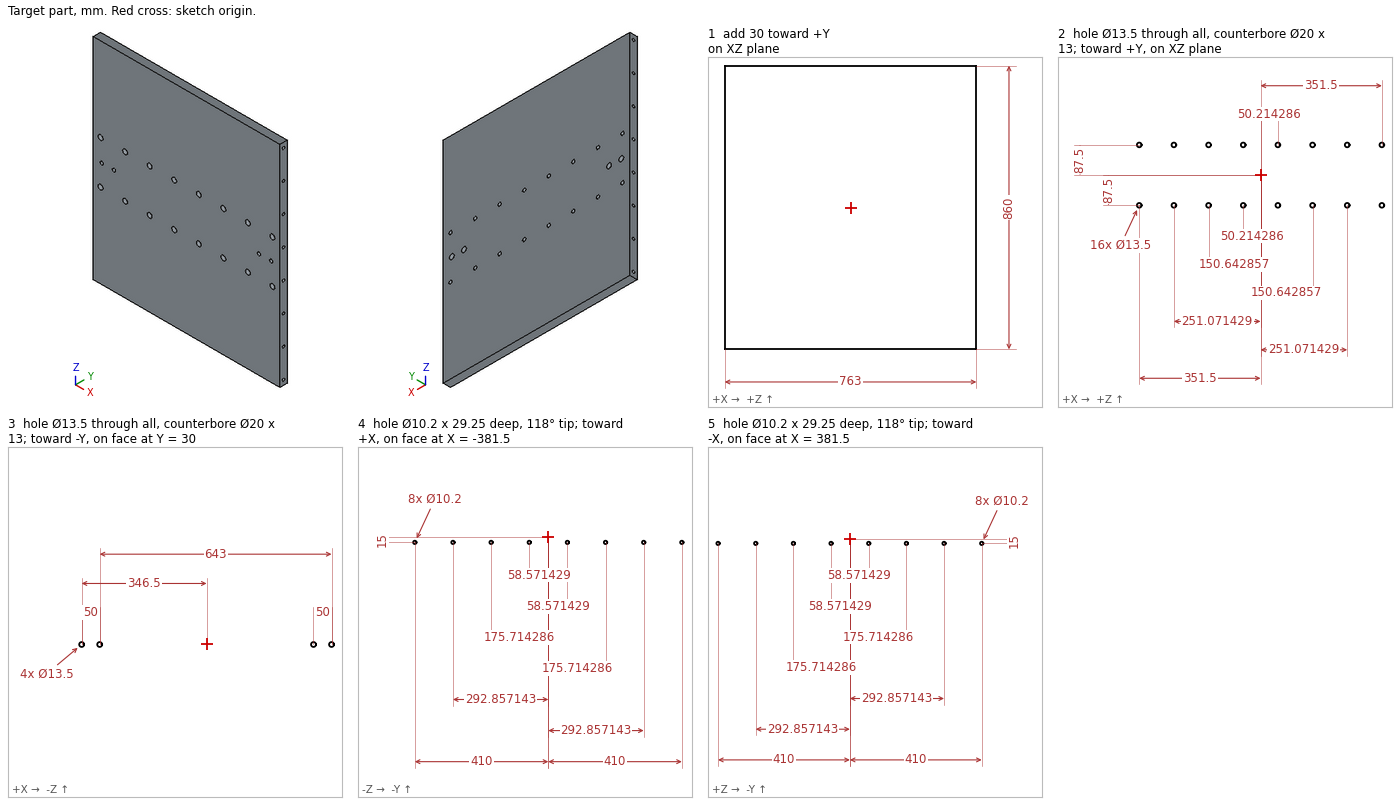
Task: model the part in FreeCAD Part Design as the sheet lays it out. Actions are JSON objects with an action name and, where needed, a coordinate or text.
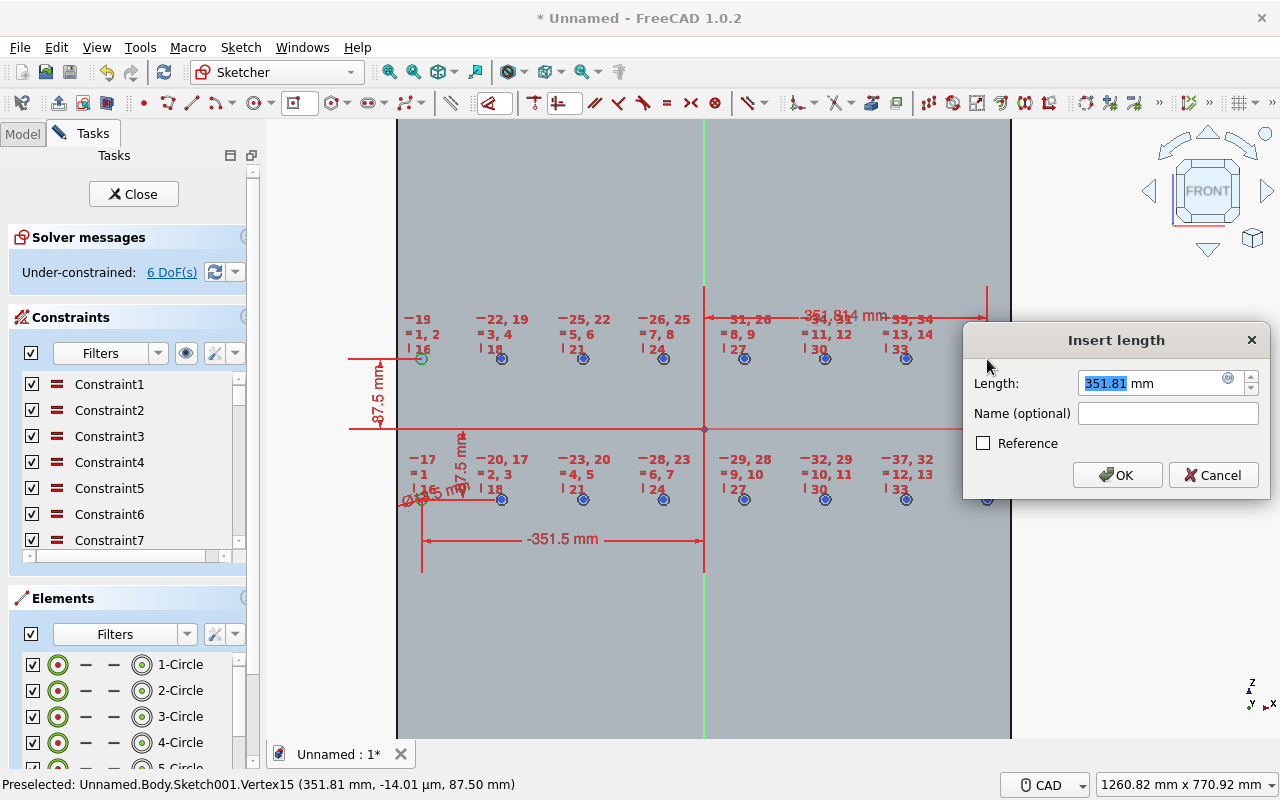
{"action": "type", "text": "351.5"}
{"action": "key", "text": "Return"}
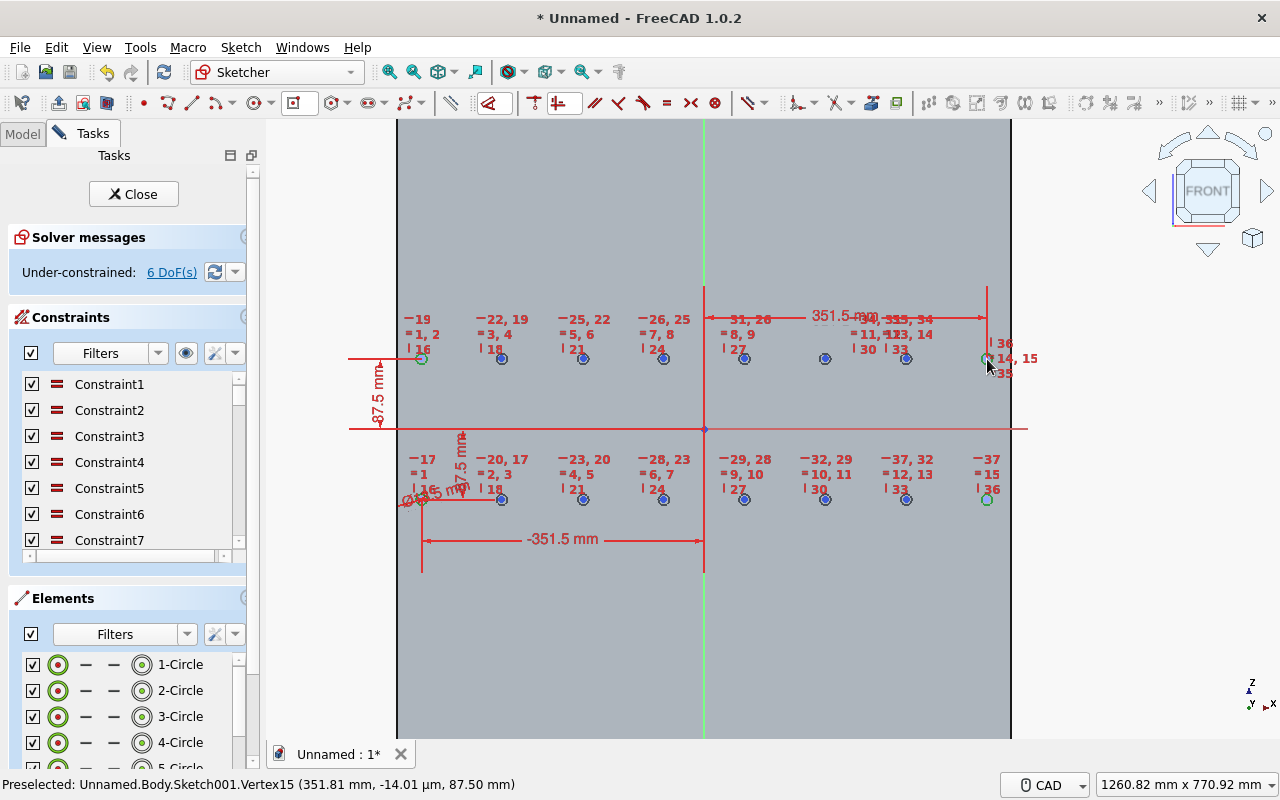
{"action": "left_click", "coordinate": [664, 500]}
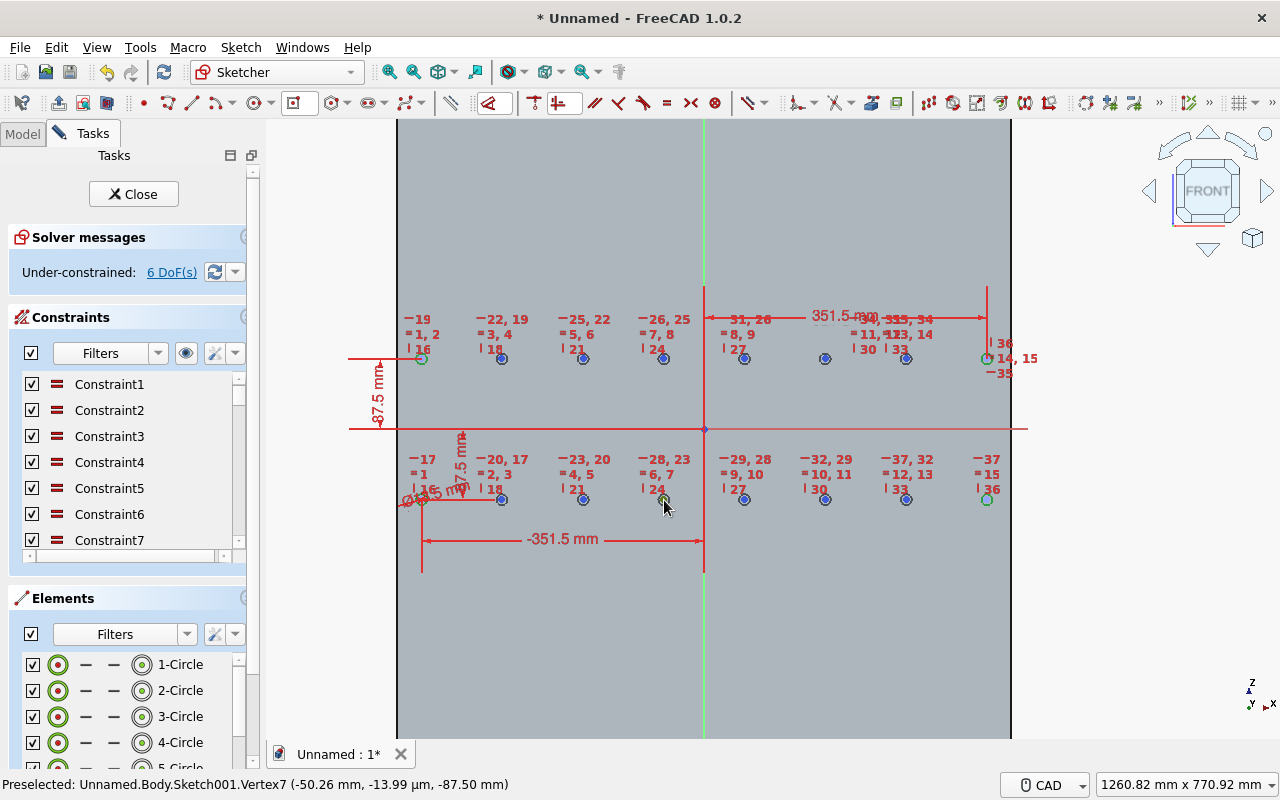
{"action": "left_click", "coordinate": [506, 104]}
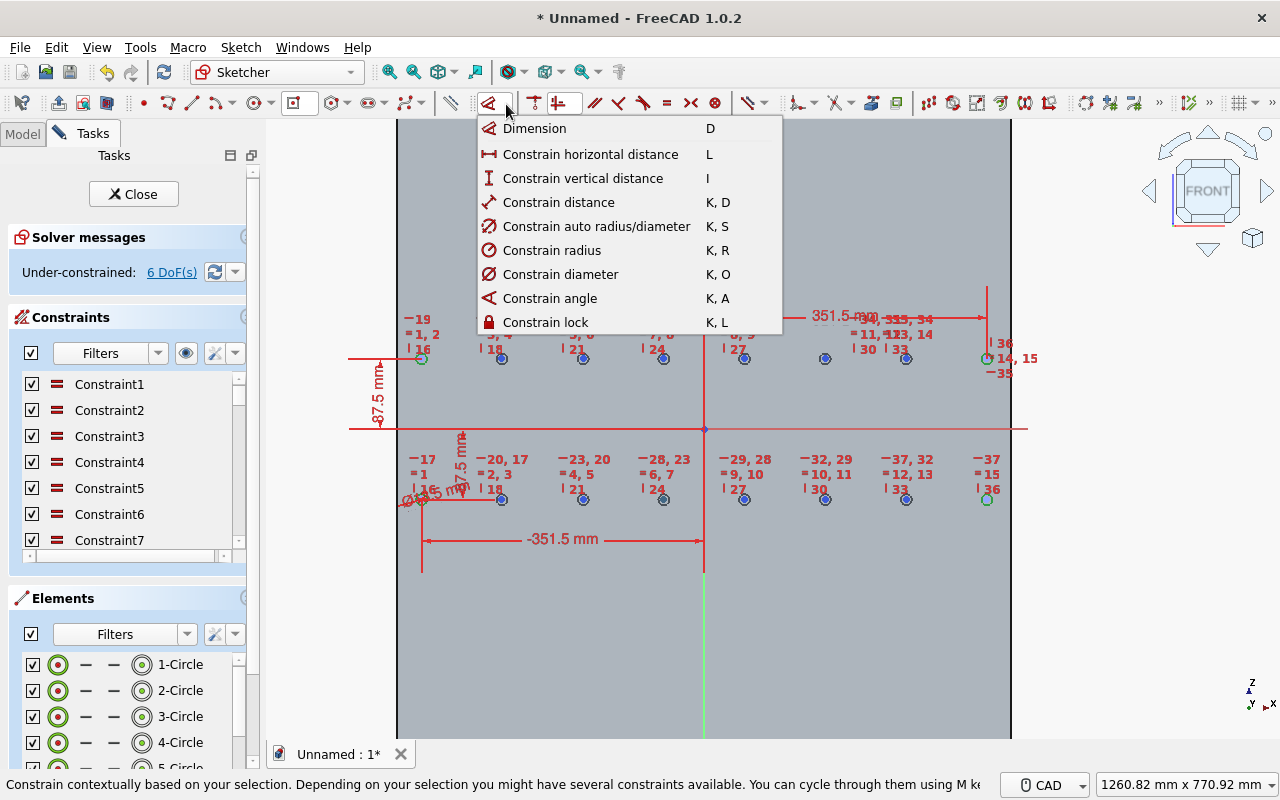
{"action": "left_click", "coordinate": [630, 154]}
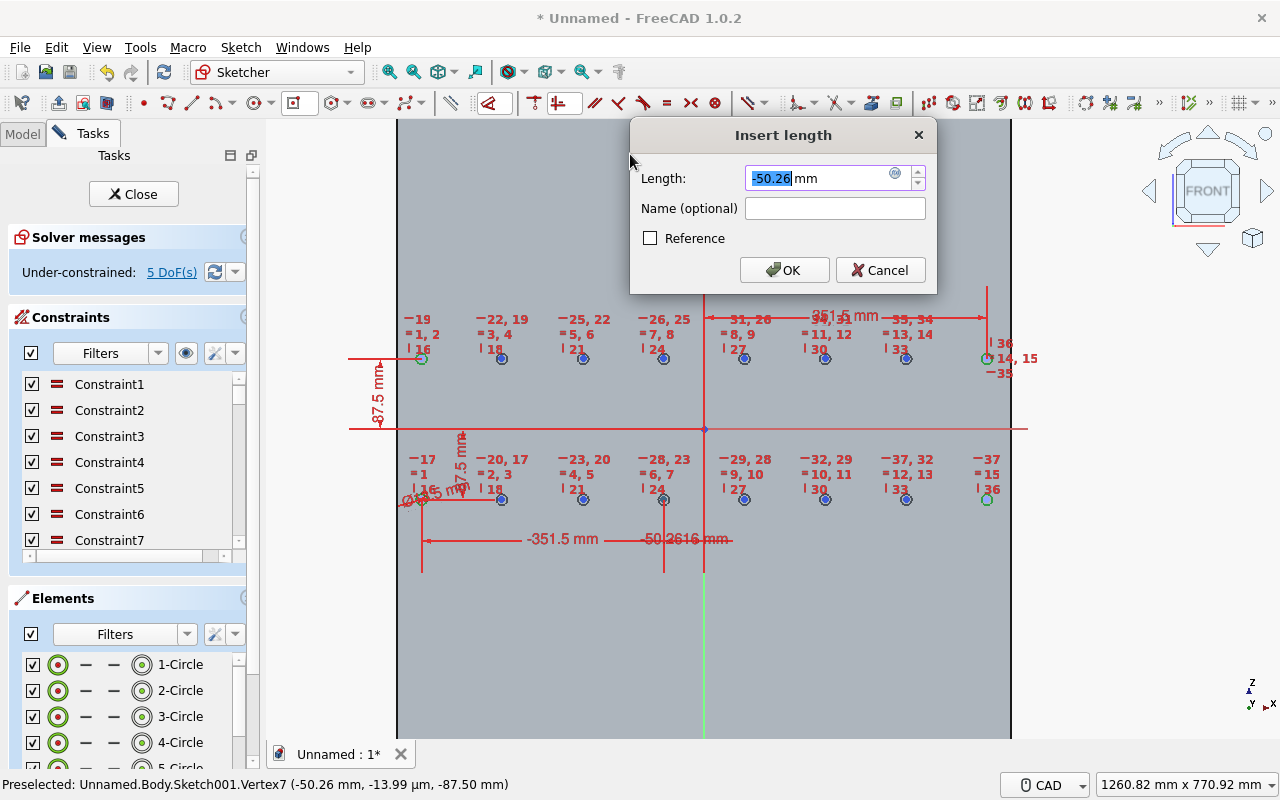
{"action": "type", "text": "-50.214286"}
{"action": "key", "text": "Return"}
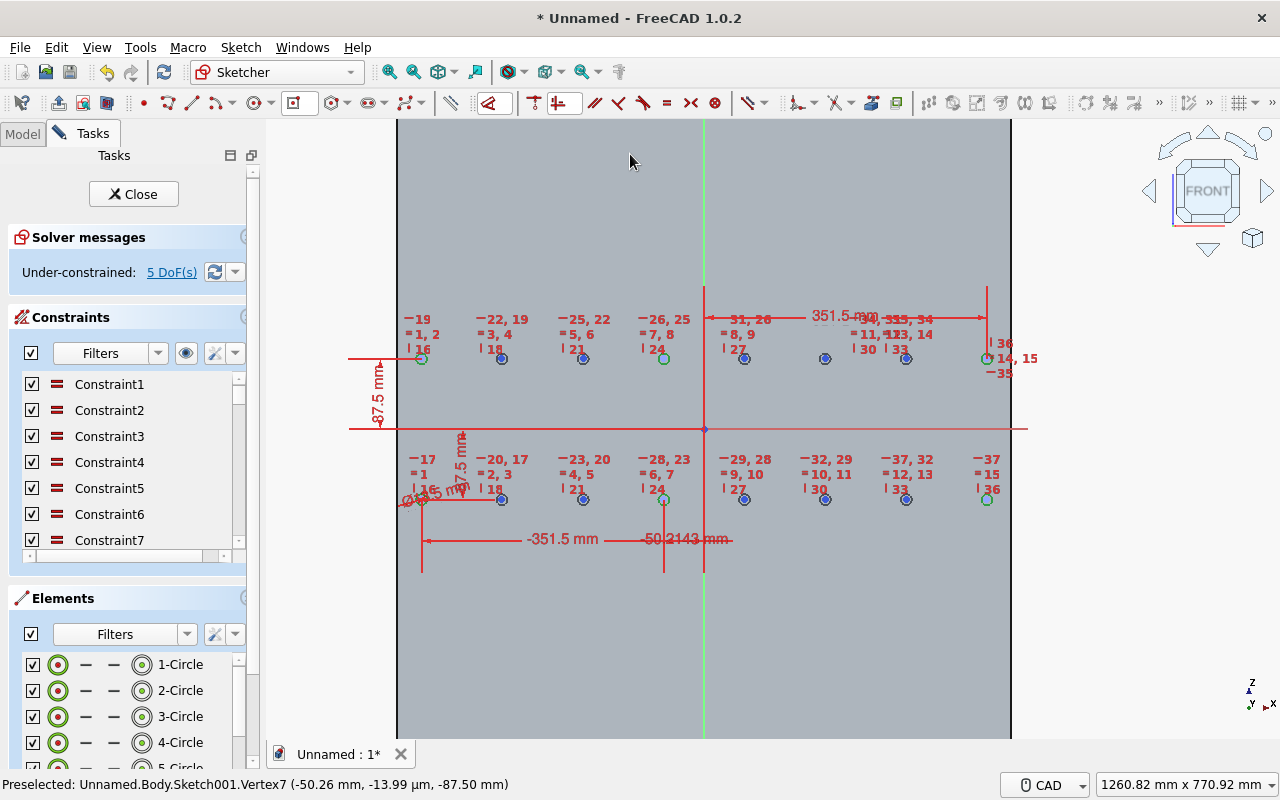
{"action": "left_click", "coordinate": [745, 359]}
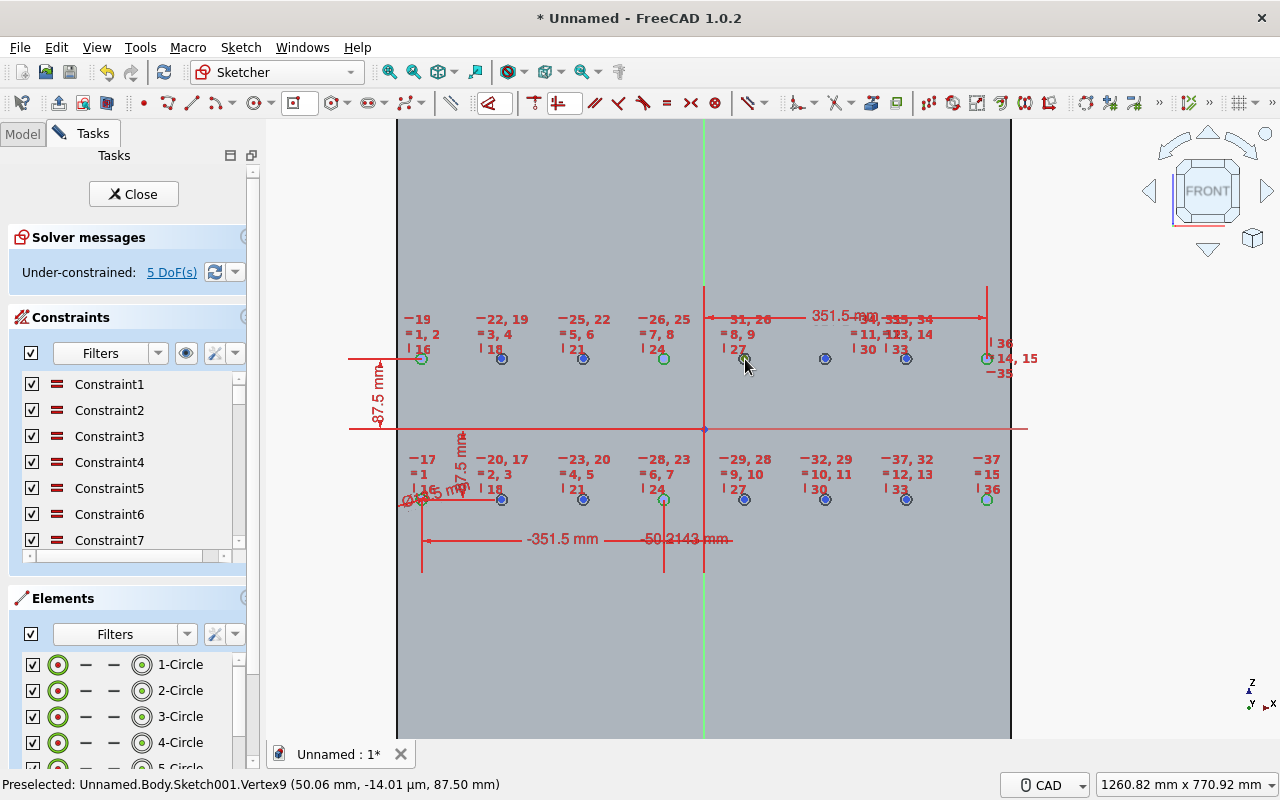
{"action": "left_click", "coordinate": [506, 104]}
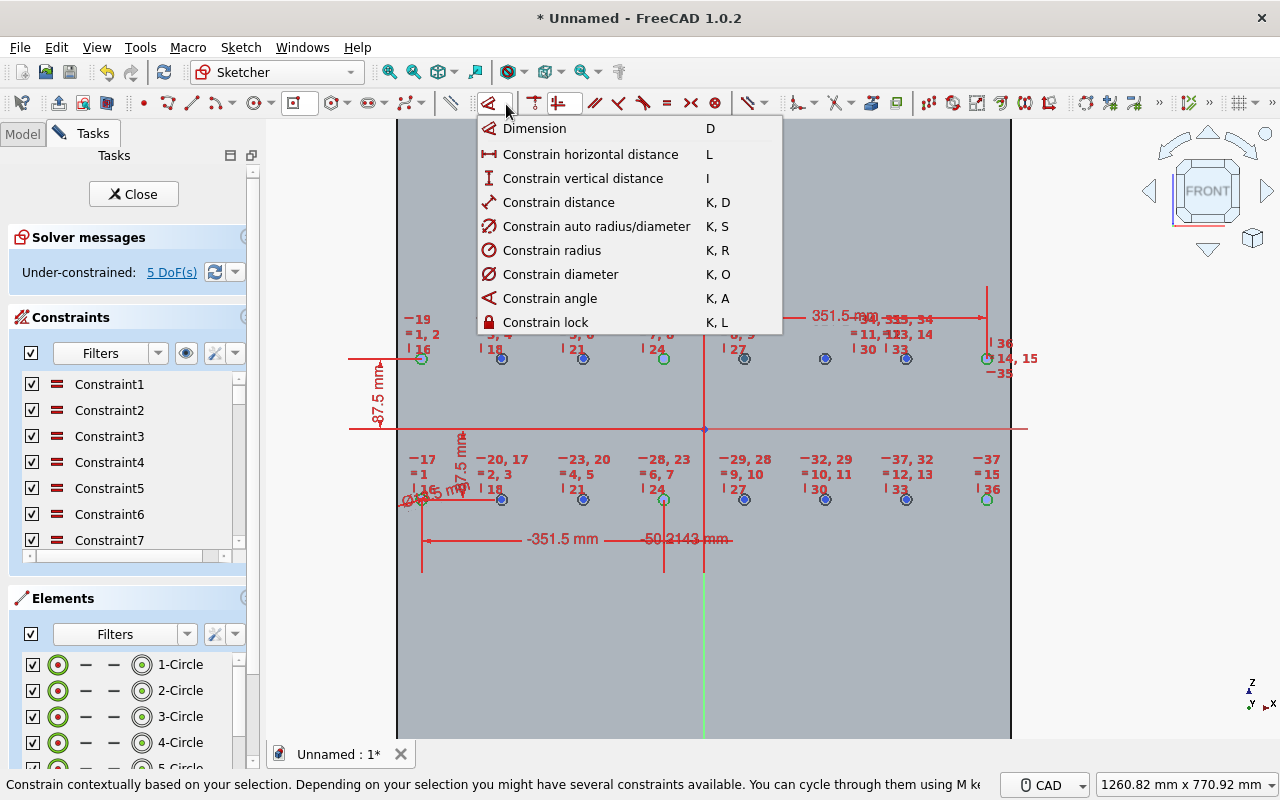
{"action": "left_click", "coordinate": [630, 154]}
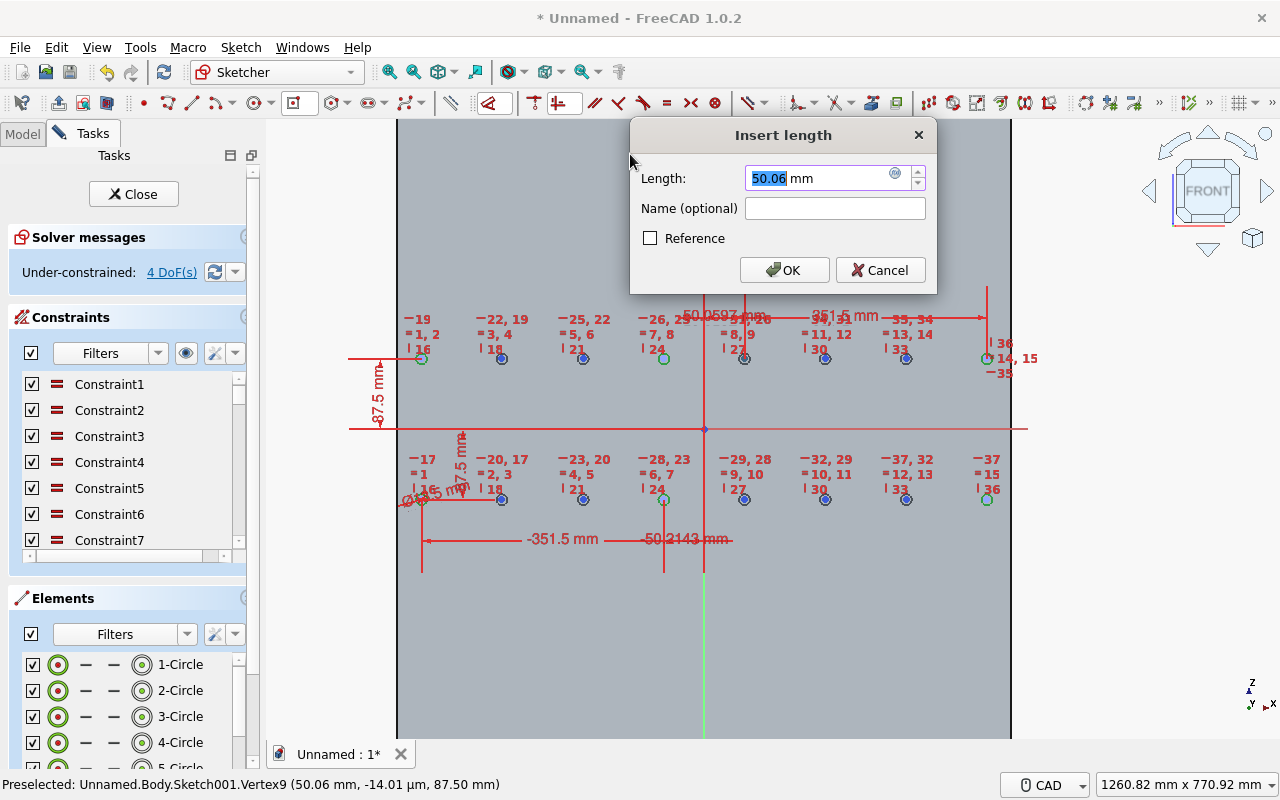
{"action": "type", "text": "50.214286"}
{"action": "key", "text": "Return"}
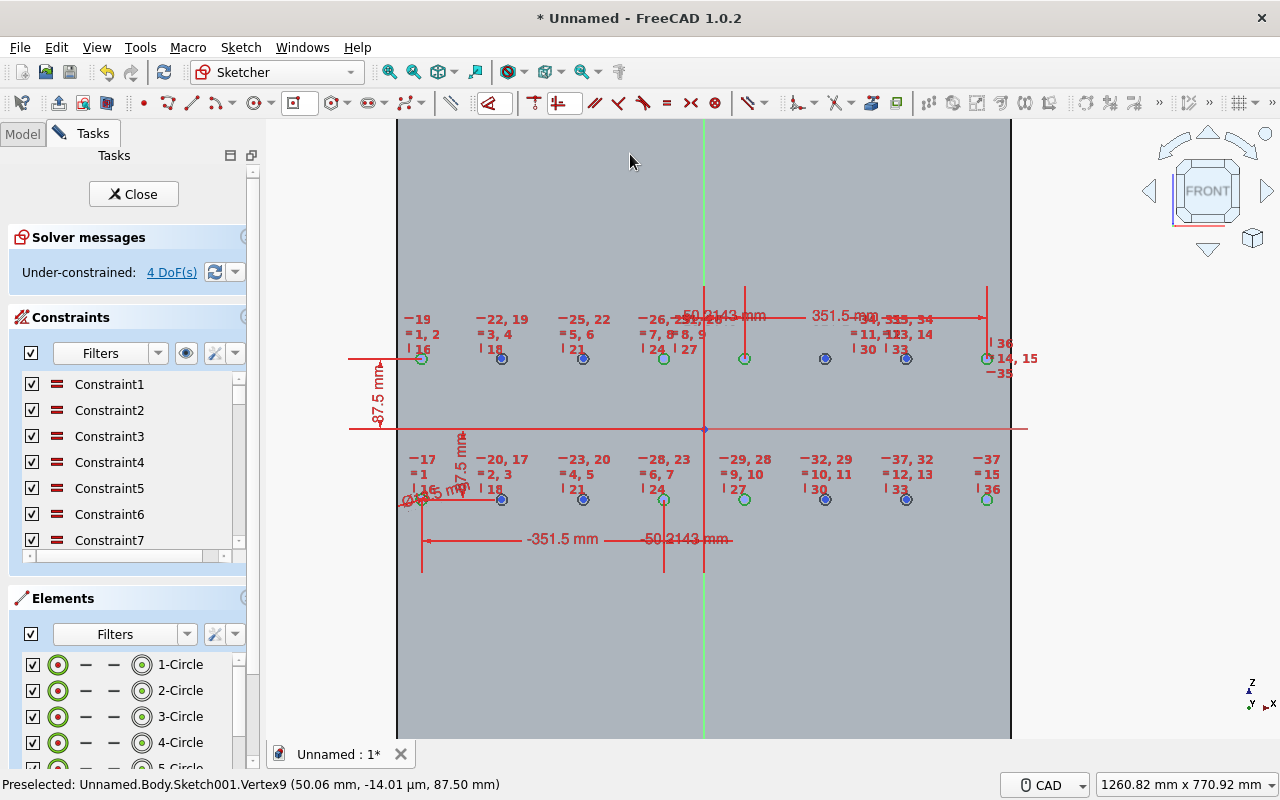
{"action": "left_click", "coordinate": [502, 500]}